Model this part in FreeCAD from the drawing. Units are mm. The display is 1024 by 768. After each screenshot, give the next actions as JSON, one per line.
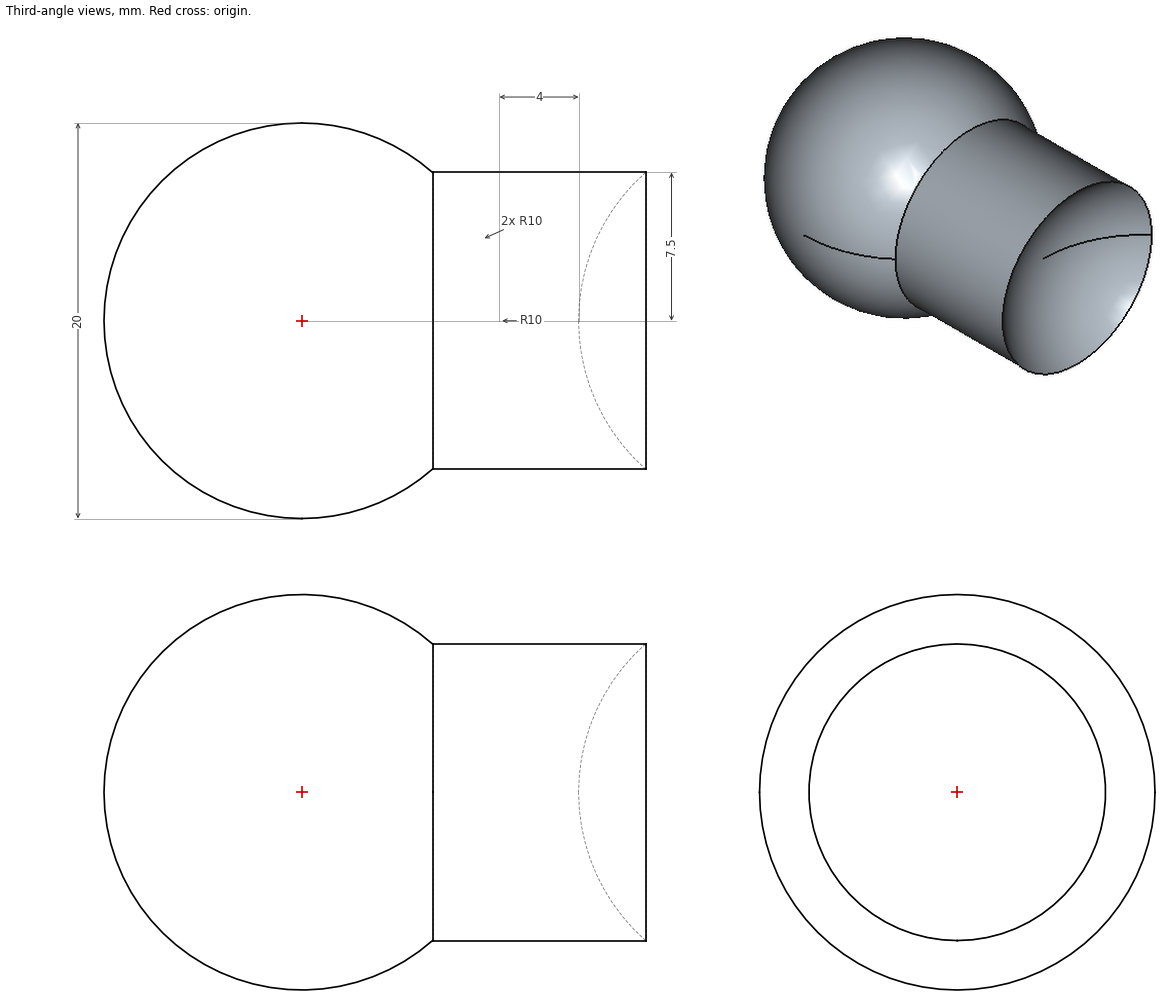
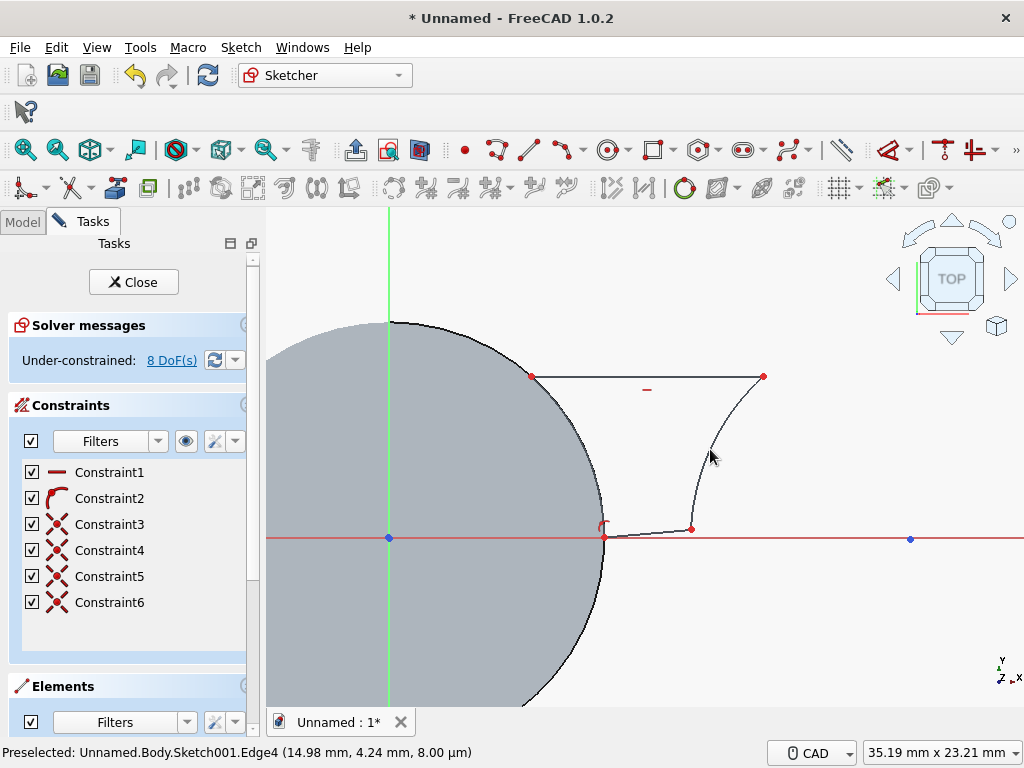
{"action": "left_click", "coordinate": [630, 535]}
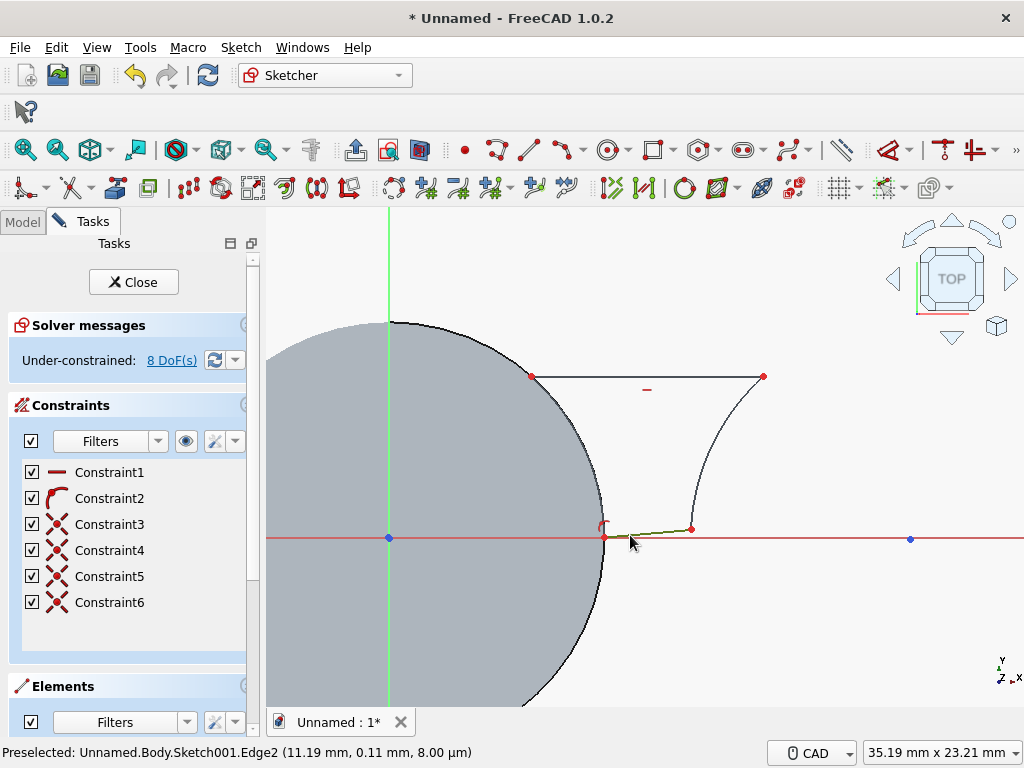
{"action": "key", "text": "h"}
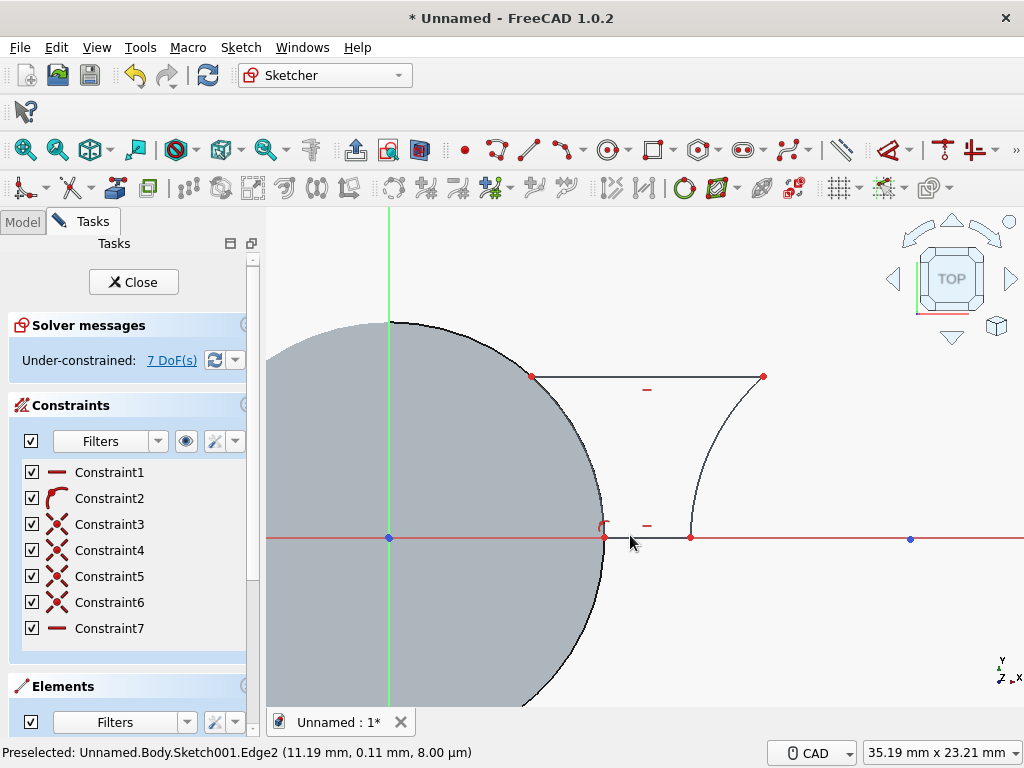
{"action": "left_click_drag", "start_coordinate": [379, 528], "coordinate": [399, 548]}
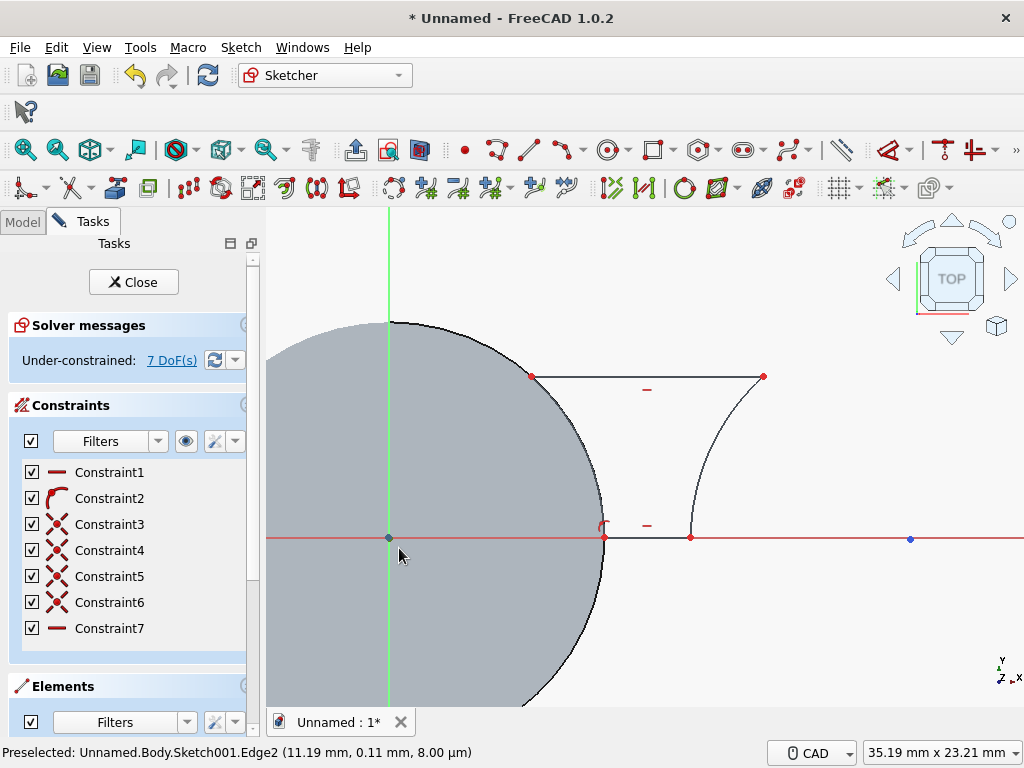
{"action": "left_click", "coordinate": [944, 150]}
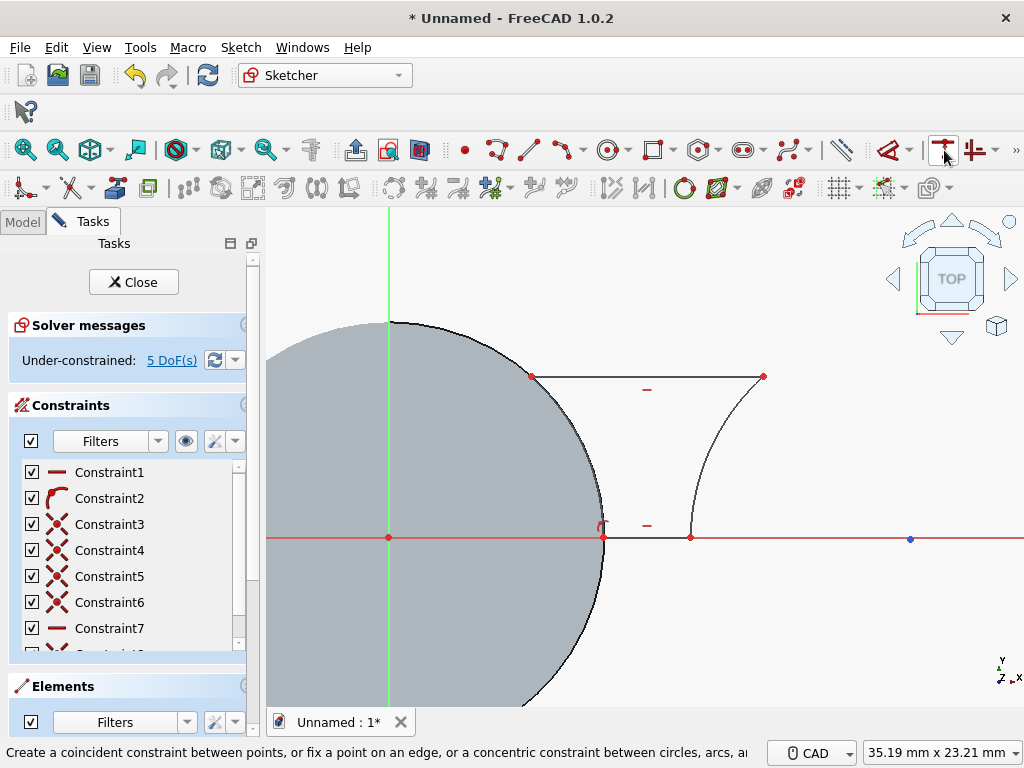
{"action": "left_click", "coordinate": [596, 484]}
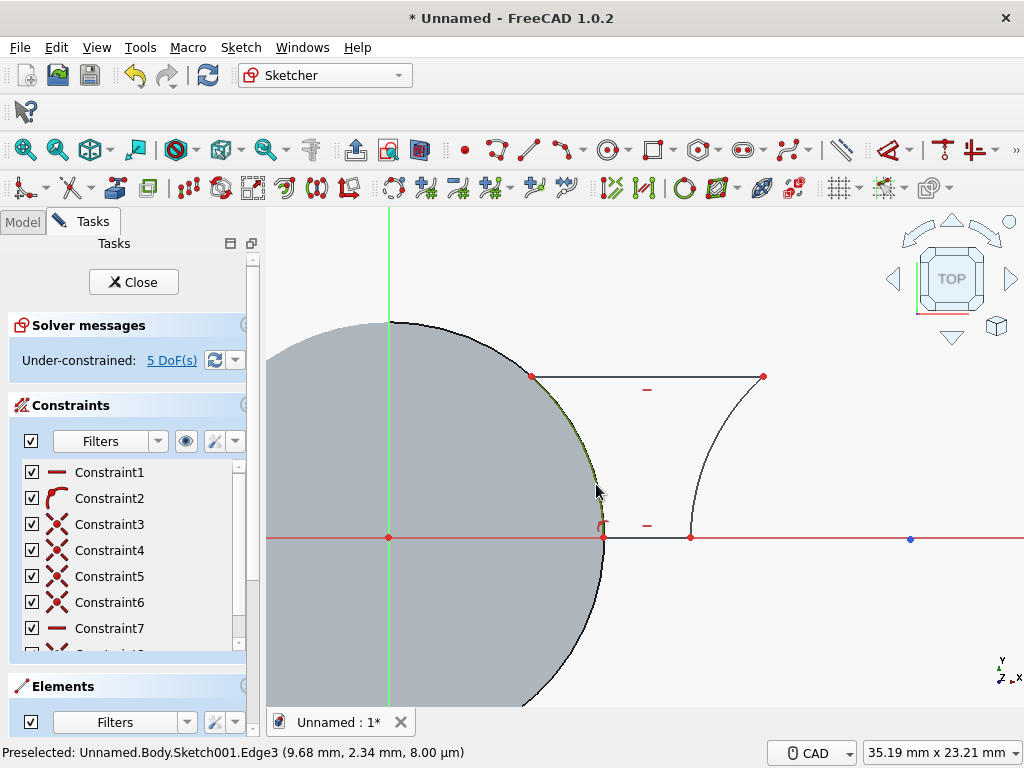
{"action": "left_click", "coordinate": [728, 418]}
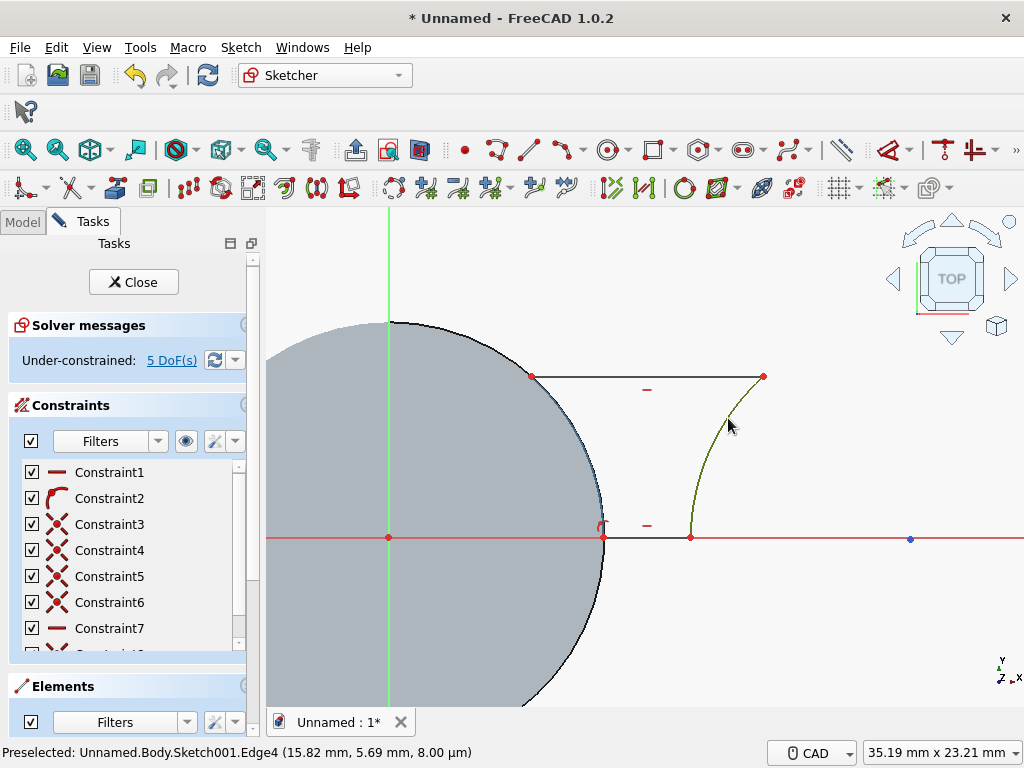
{"action": "key", "text": "e"}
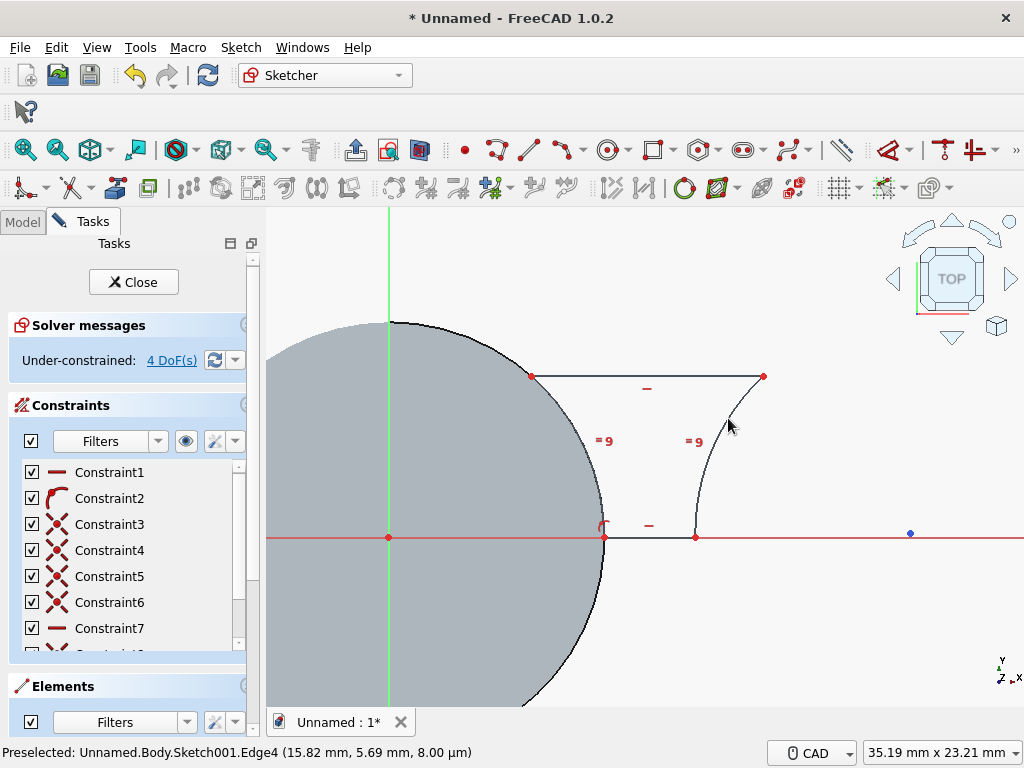
{"action": "scroll", "coordinate": [294, 458], "scroll_direction": "down", "scroll_amount": 1}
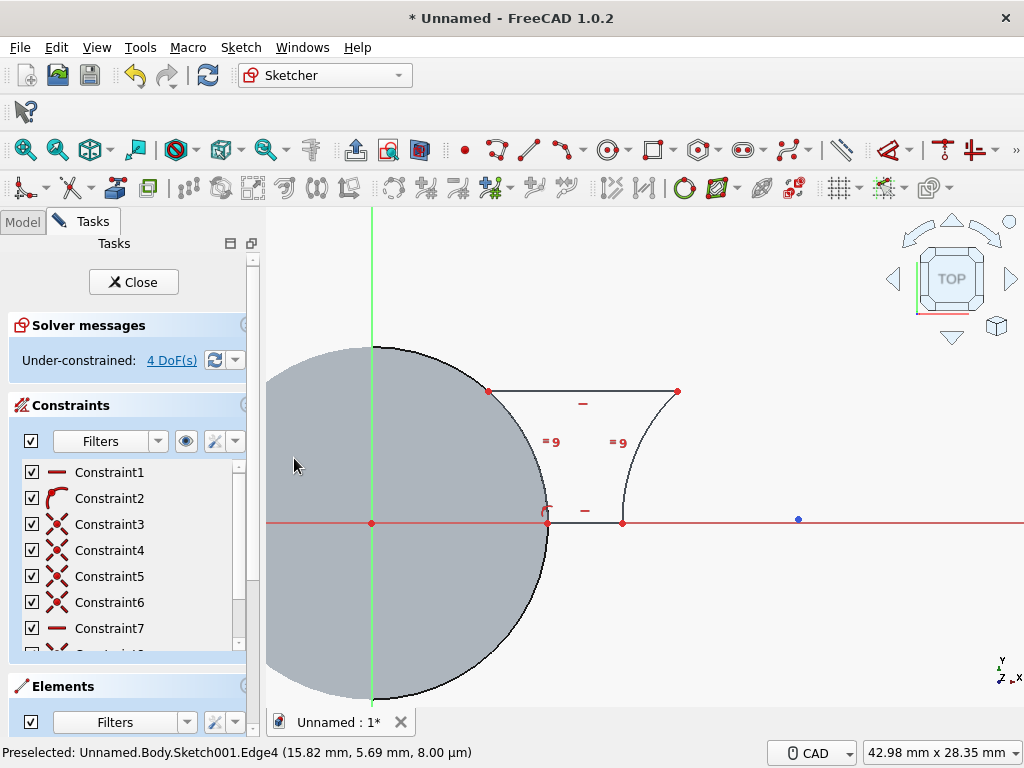
{"action": "left_click", "coordinate": [799, 520]}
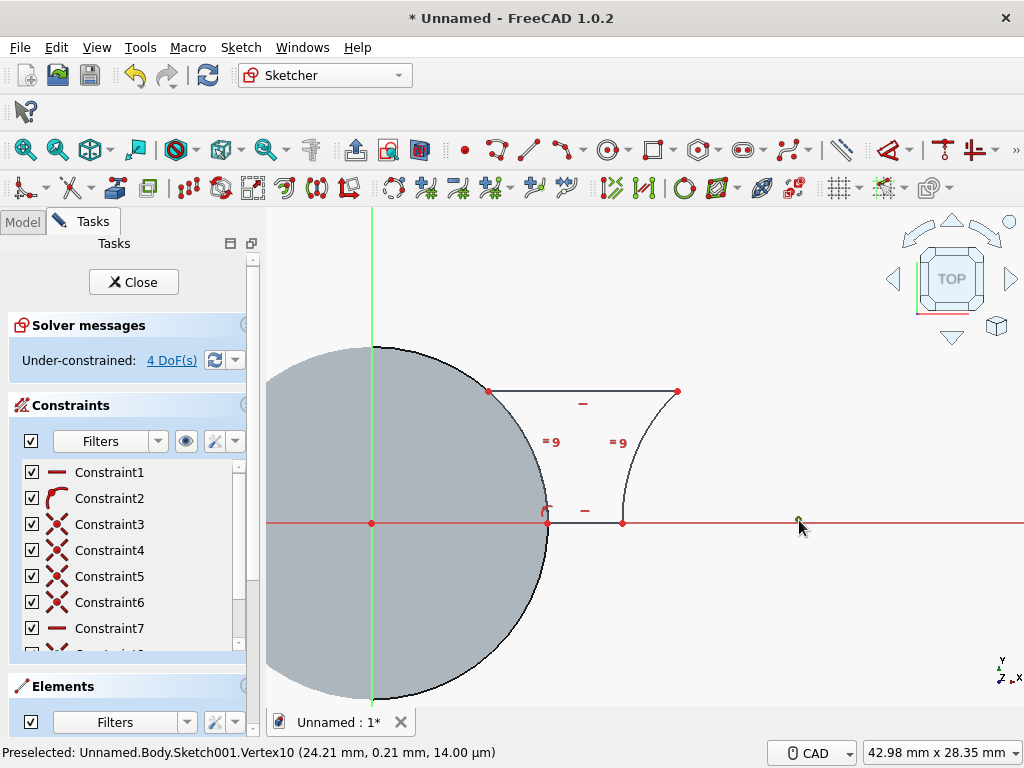
{"action": "left_click", "coordinate": [334, 523]}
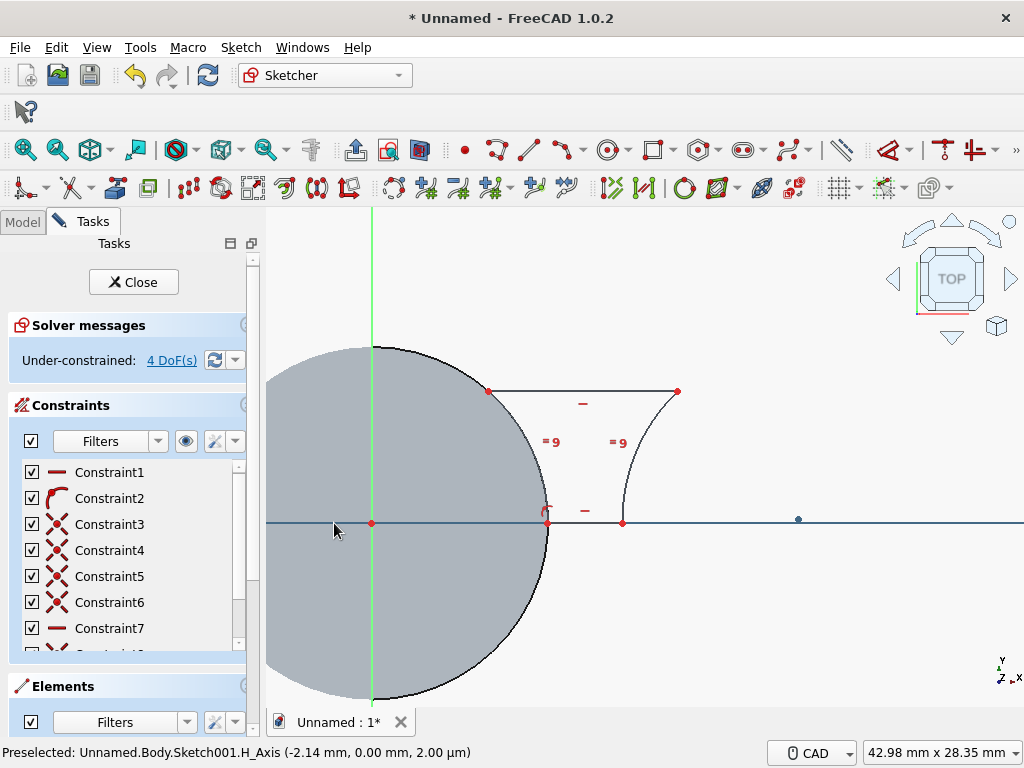
{"action": "key", "text": "c"}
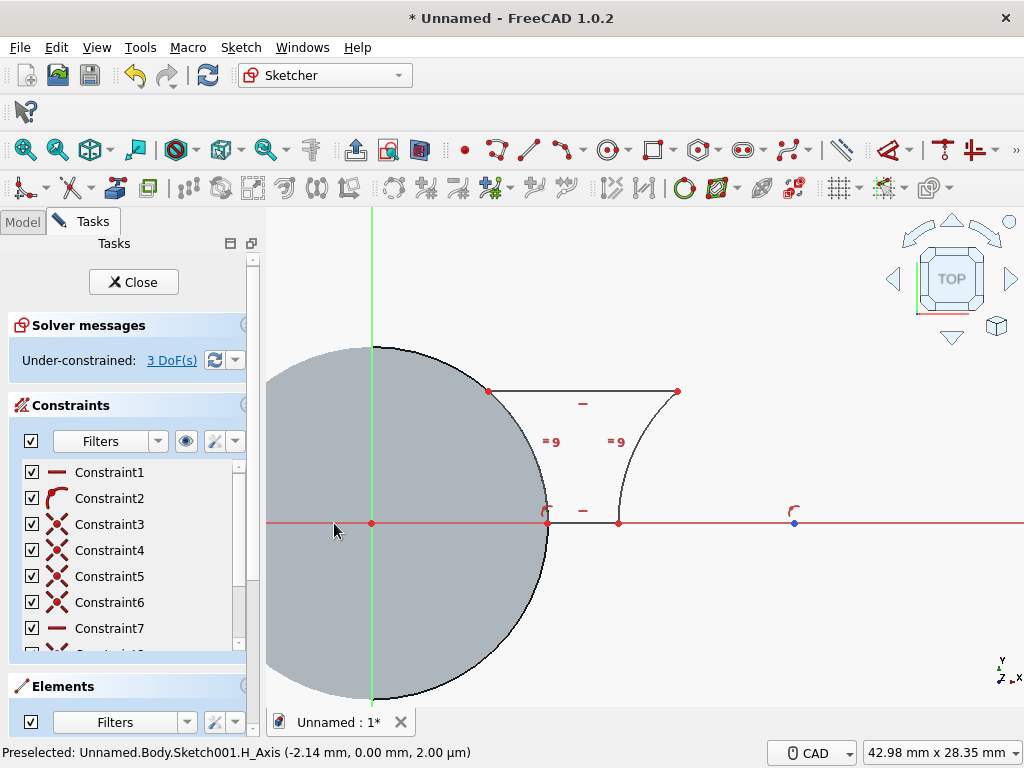
{"action": "key", "text": "d"}